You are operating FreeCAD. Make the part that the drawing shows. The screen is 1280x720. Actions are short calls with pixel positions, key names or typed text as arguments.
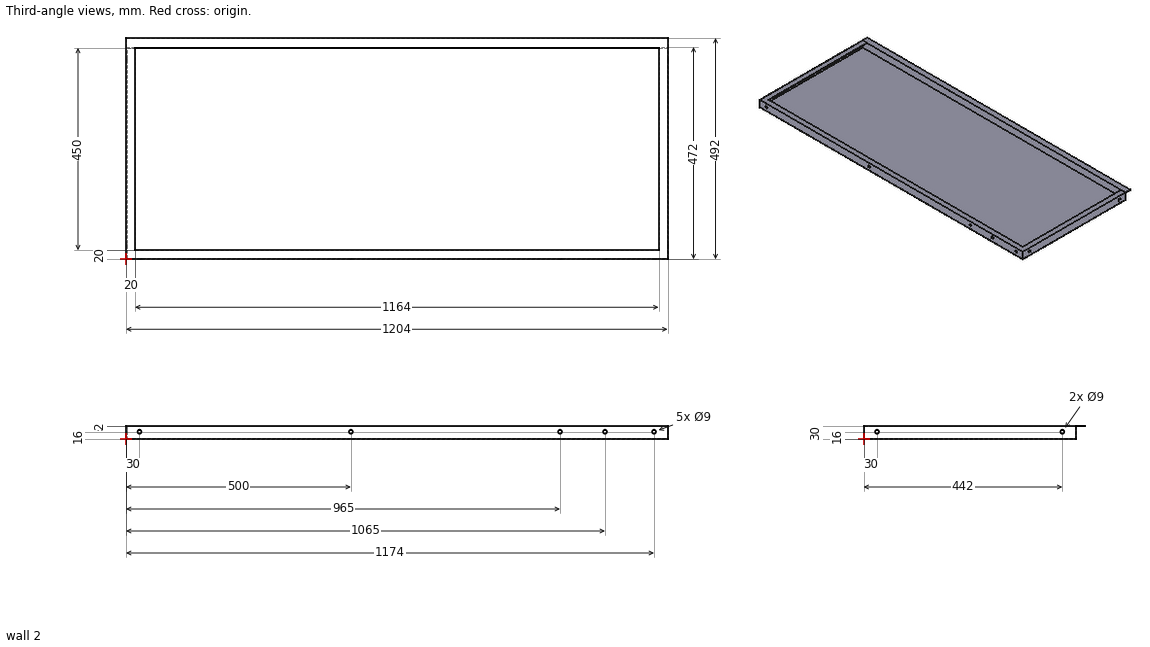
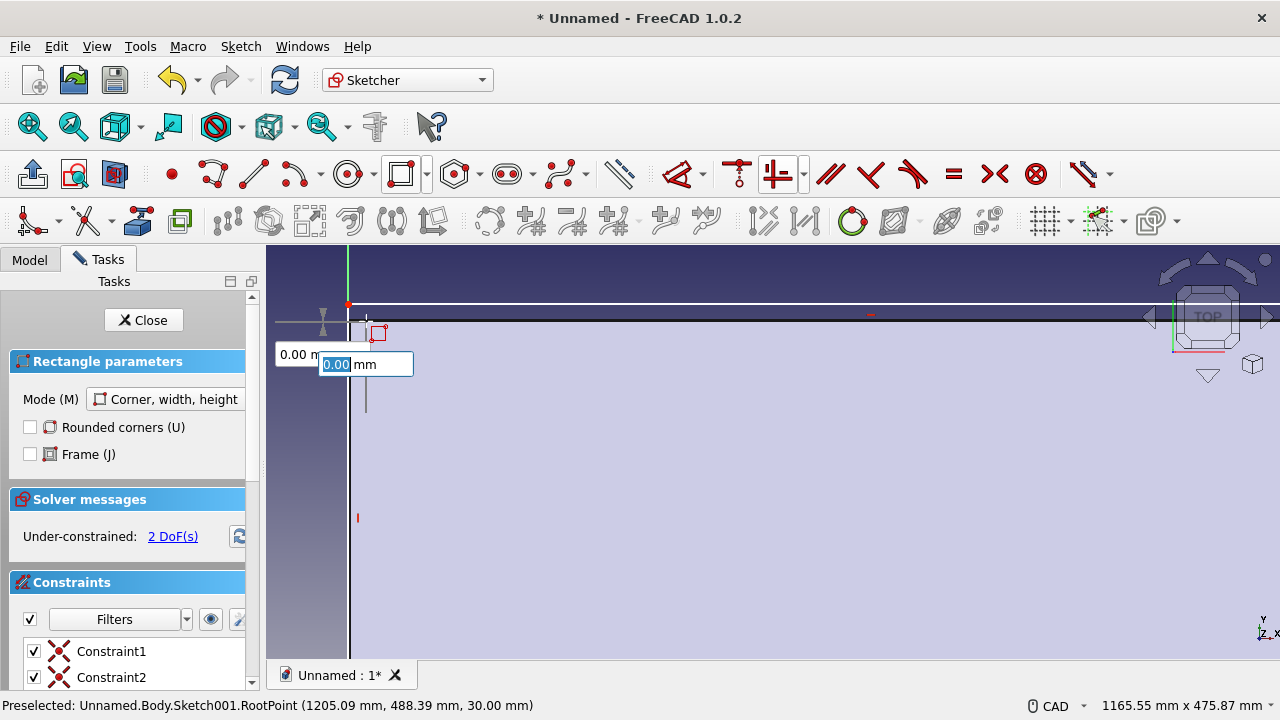
scroll(501, 374, down, 3)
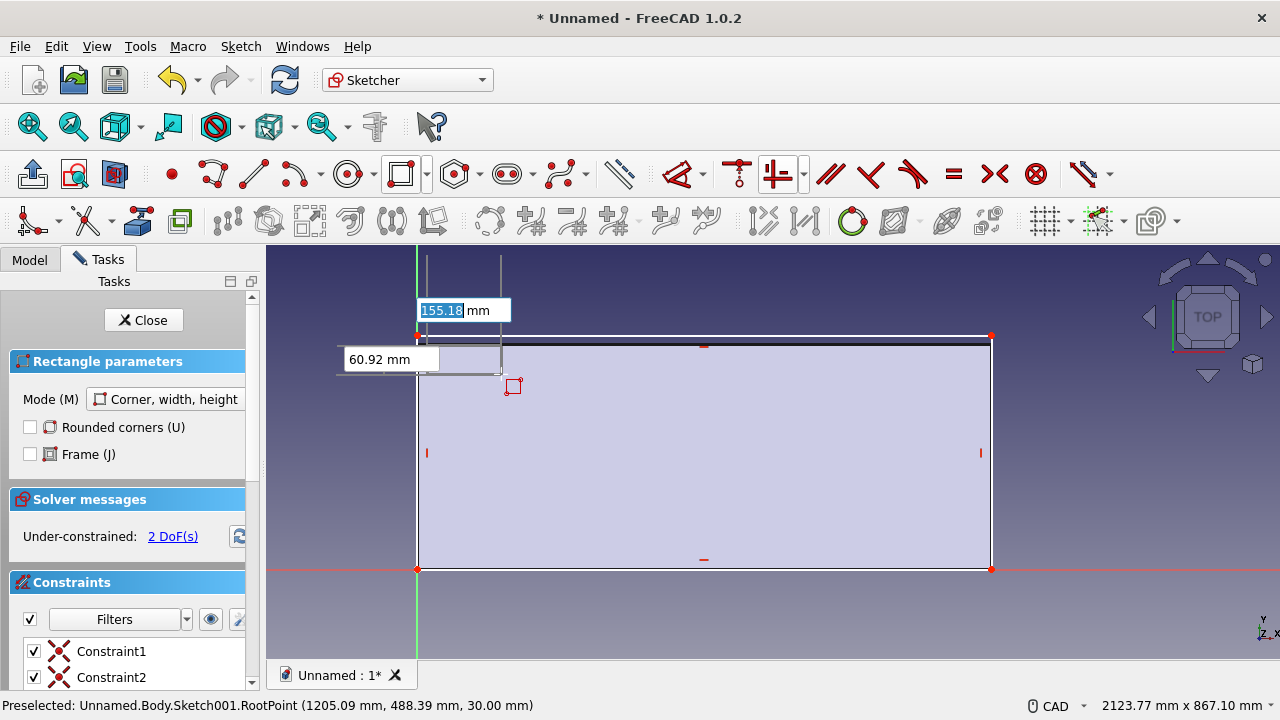
scroll(983, 560, up, 3)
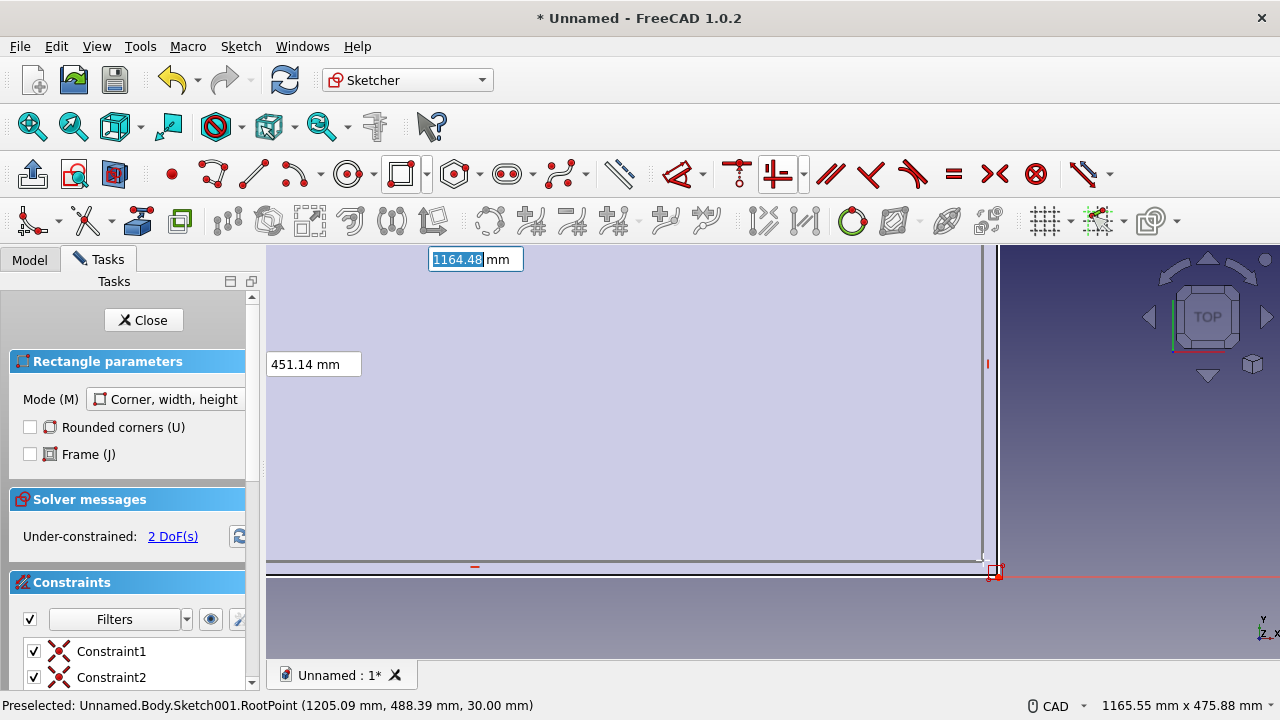
click(982, 560)
key(Escape)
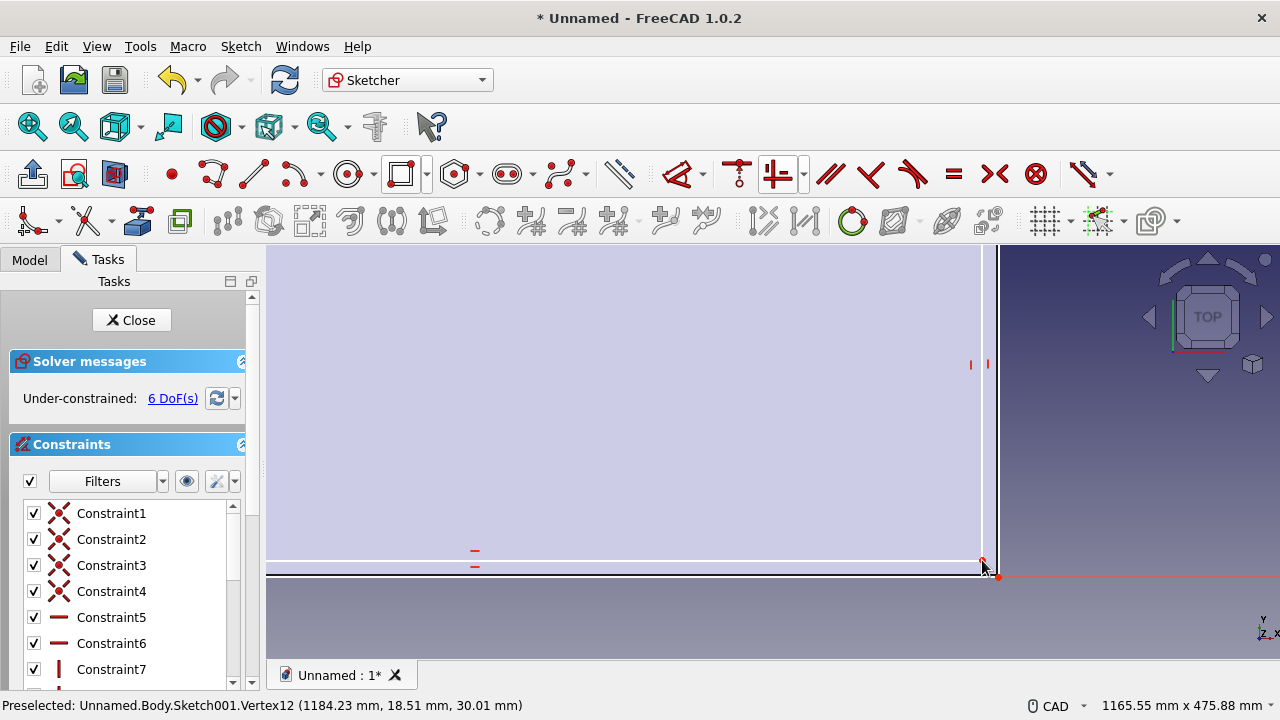
key(d)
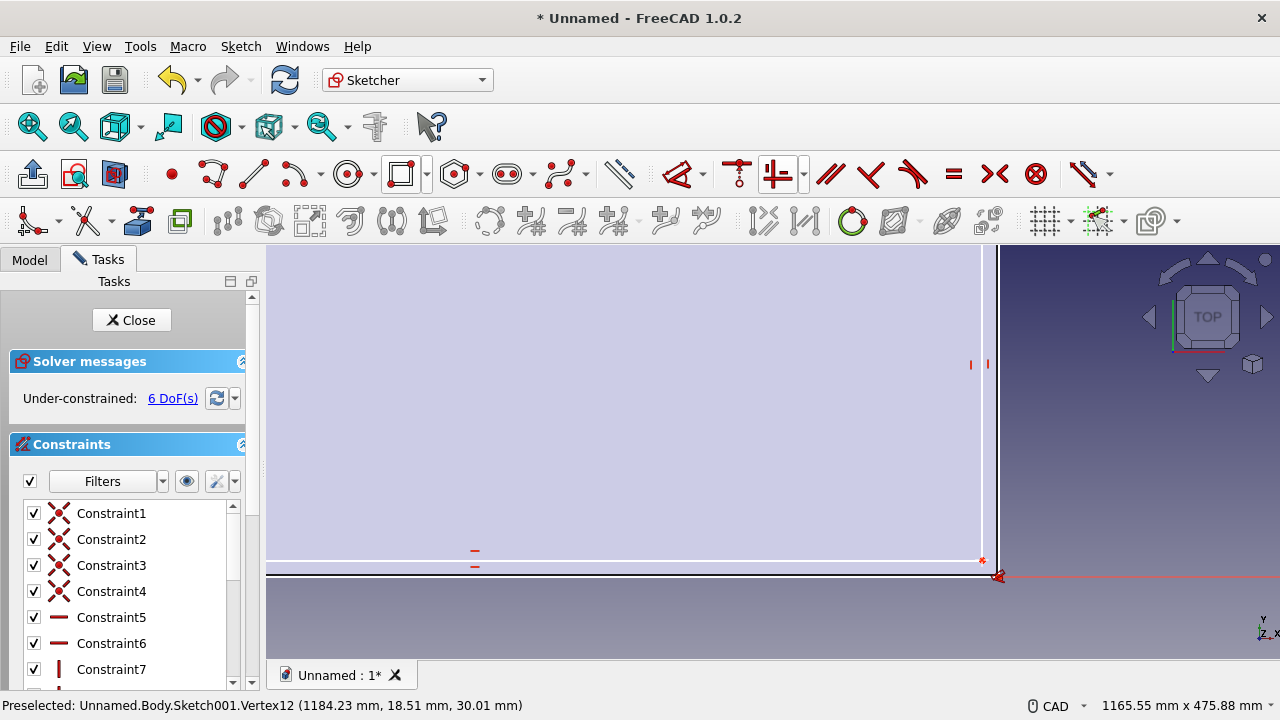
click(999, 449)
click(1033, 425)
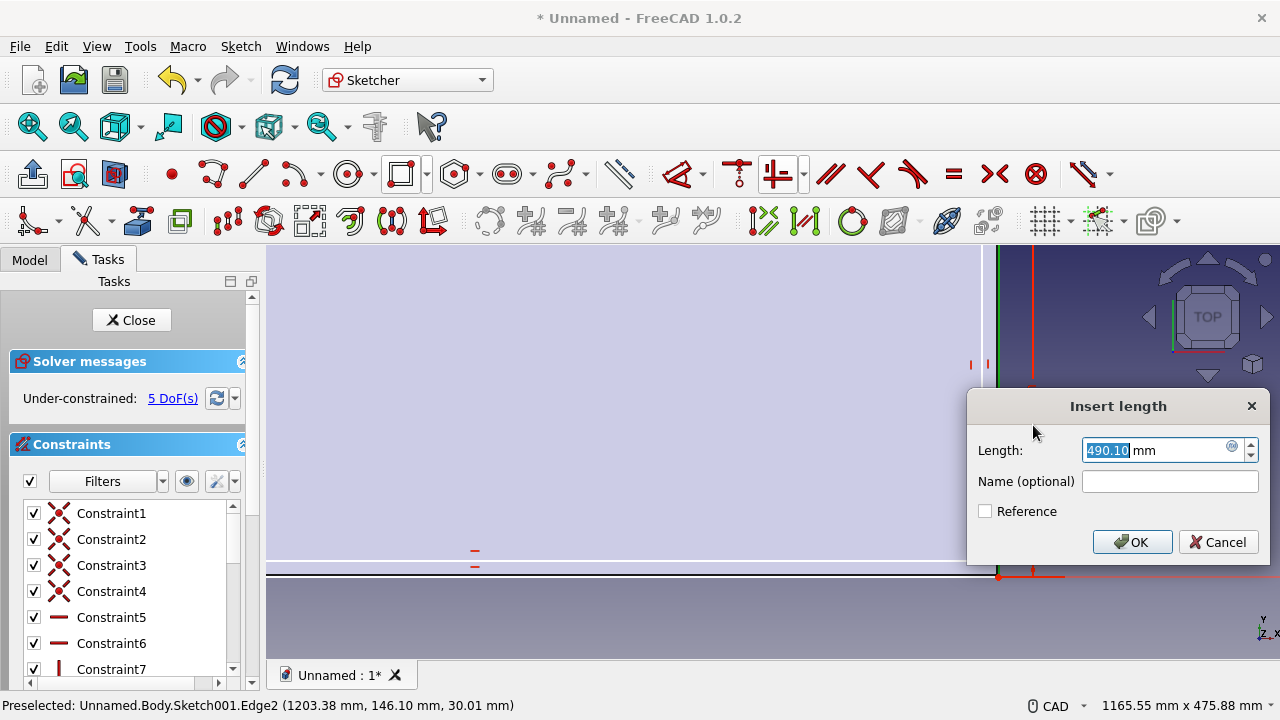
text(492)
key(Return)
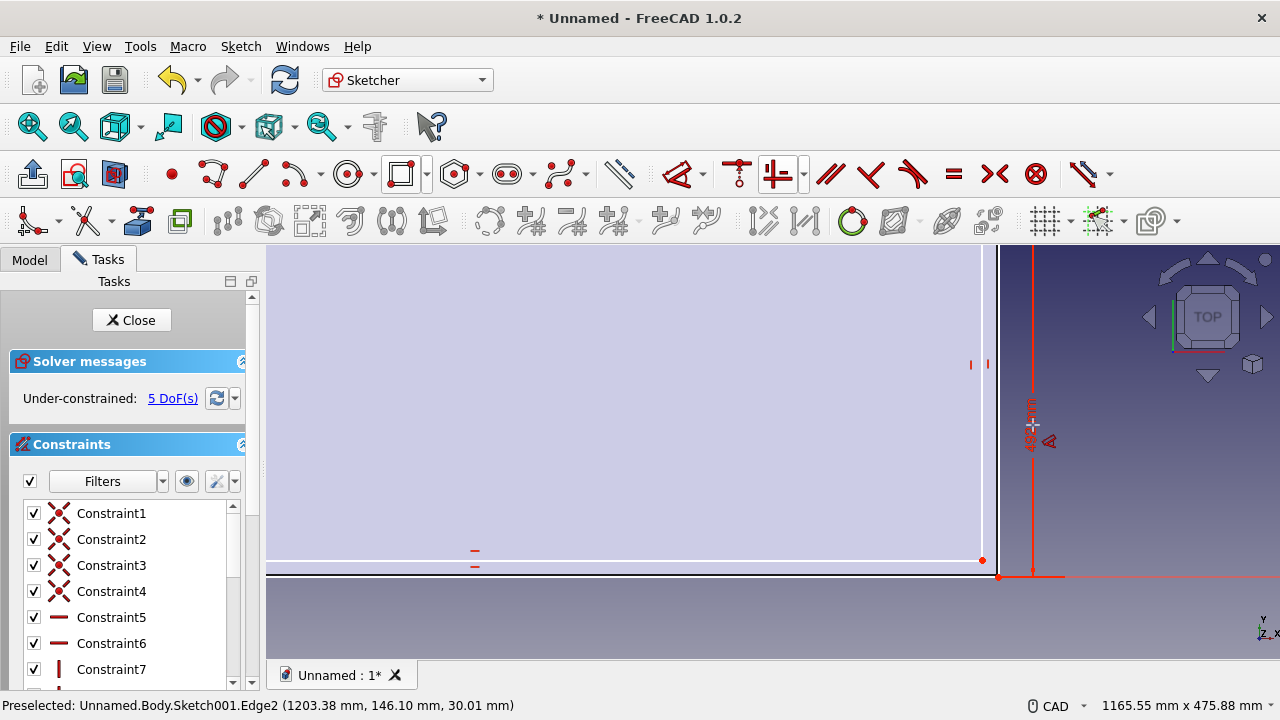
scroll(983, 560, down, 3)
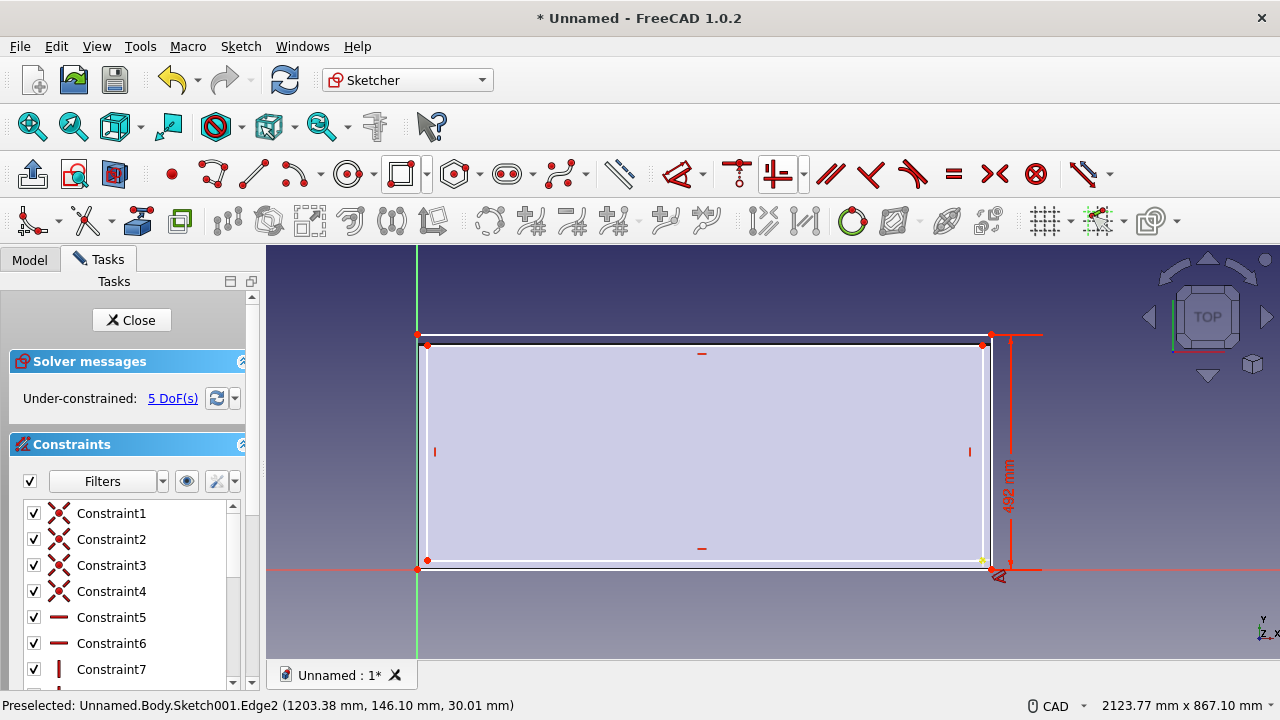
scroll(427, 410, up, 2)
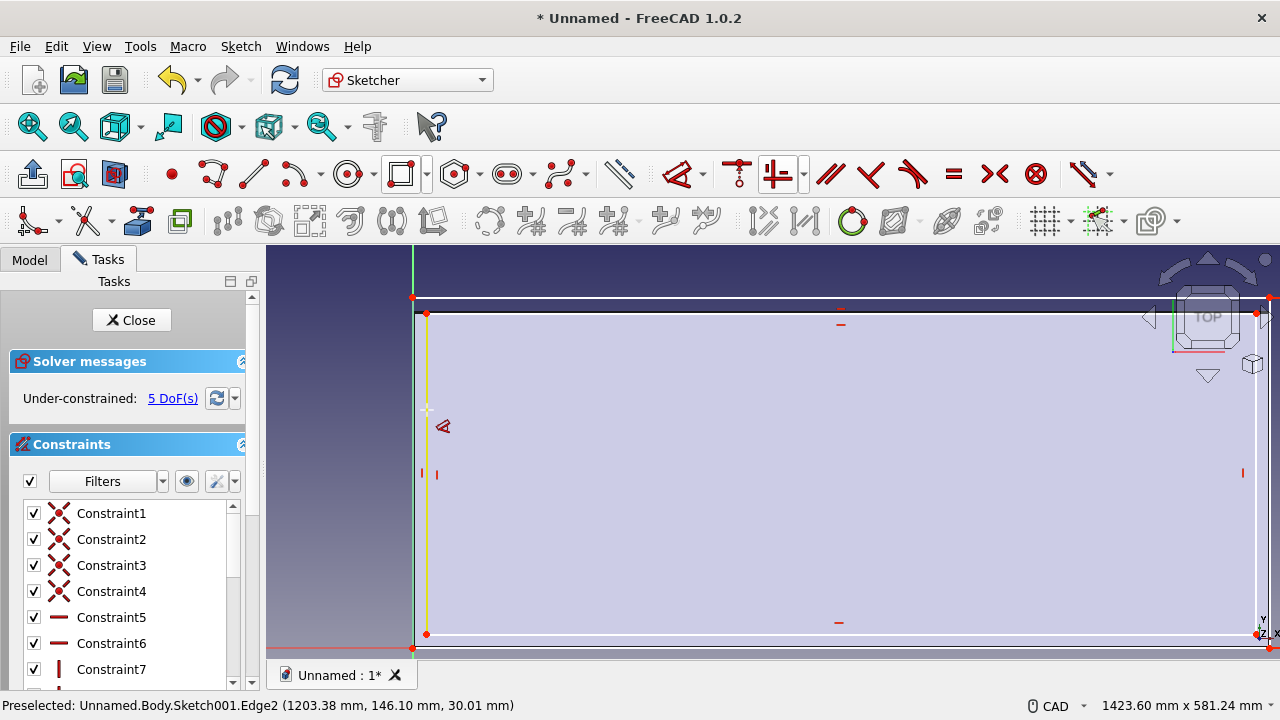
click(427, 410)
click(393, 472)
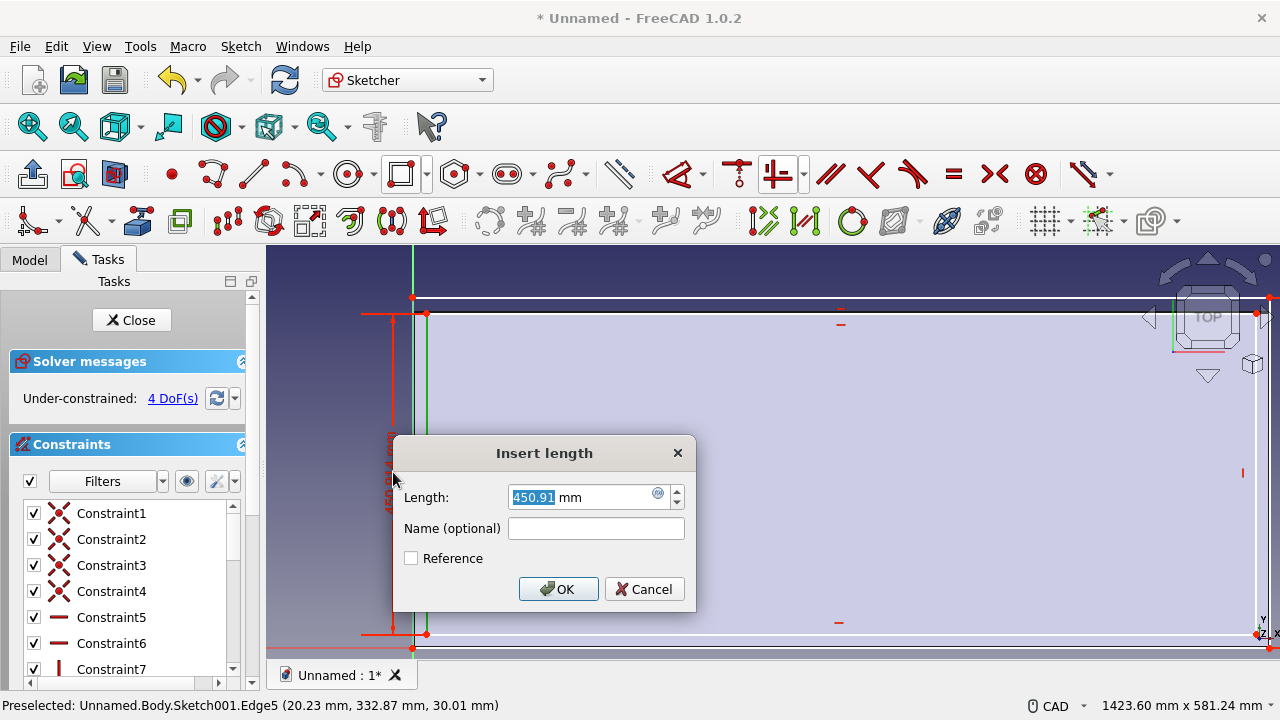
text(450)
key(Return)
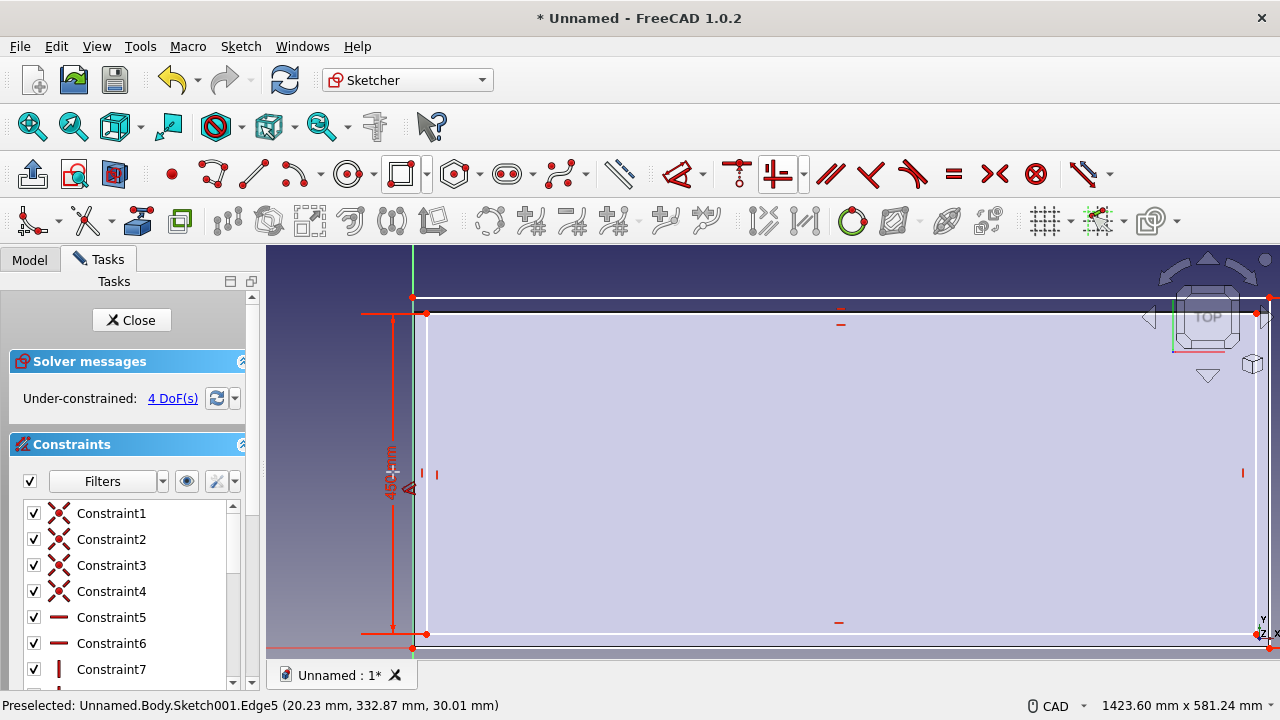
scroll(427, 314, up, 6)